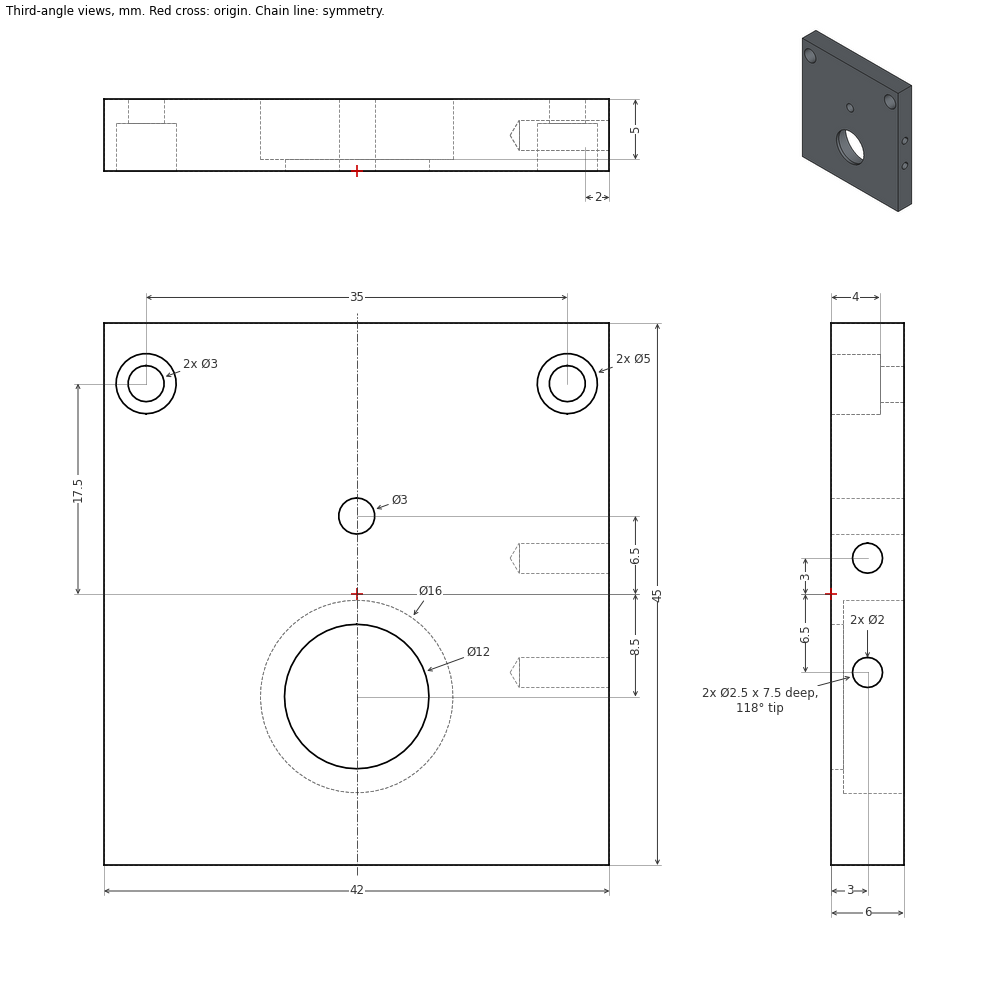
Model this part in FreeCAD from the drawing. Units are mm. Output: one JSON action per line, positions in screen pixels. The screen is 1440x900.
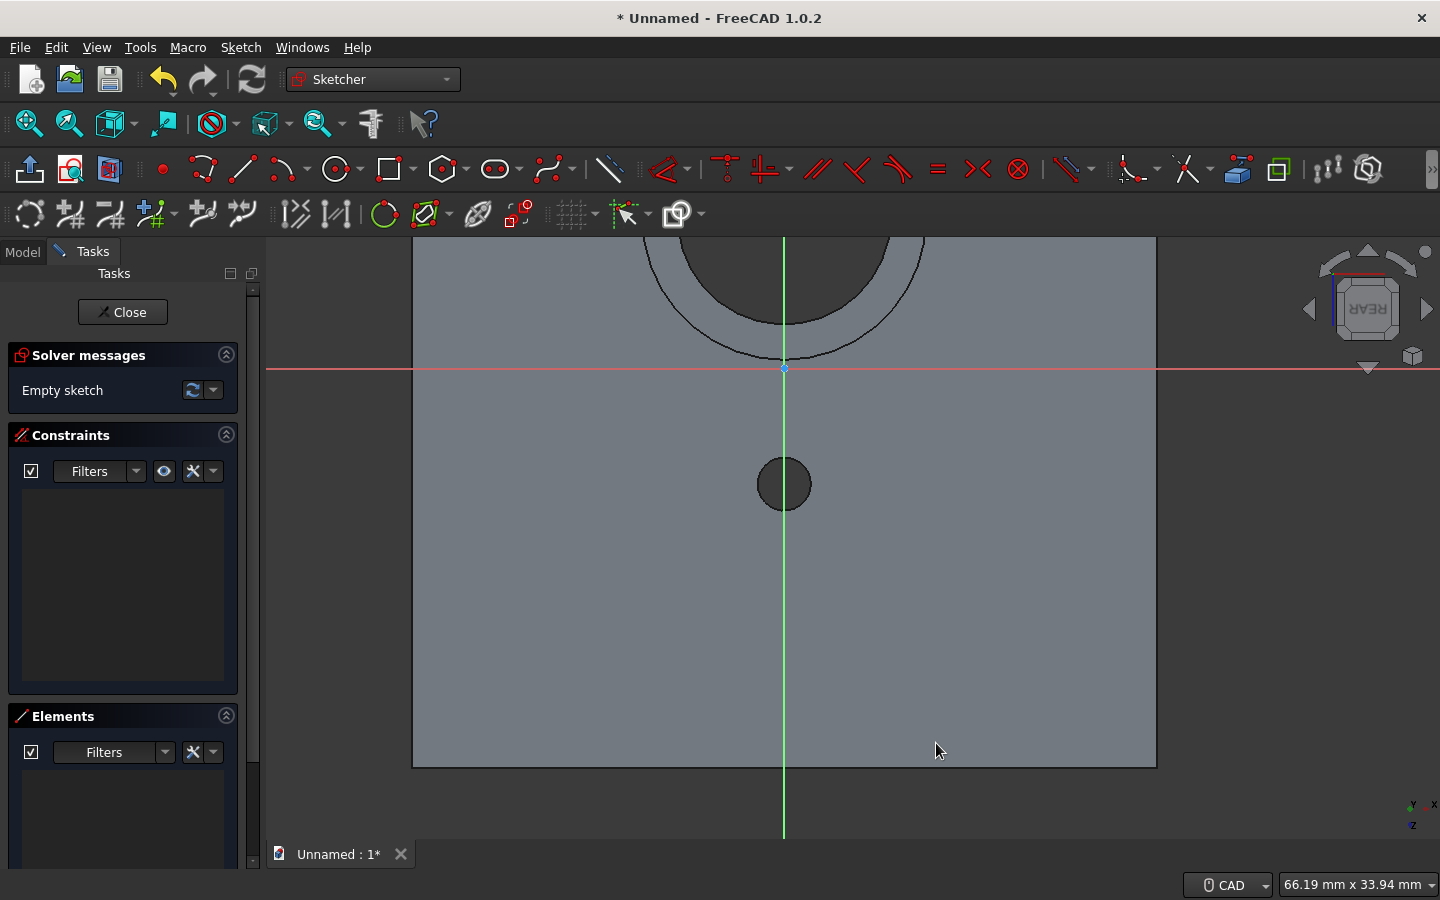
{"action": "key", "text": "g c"}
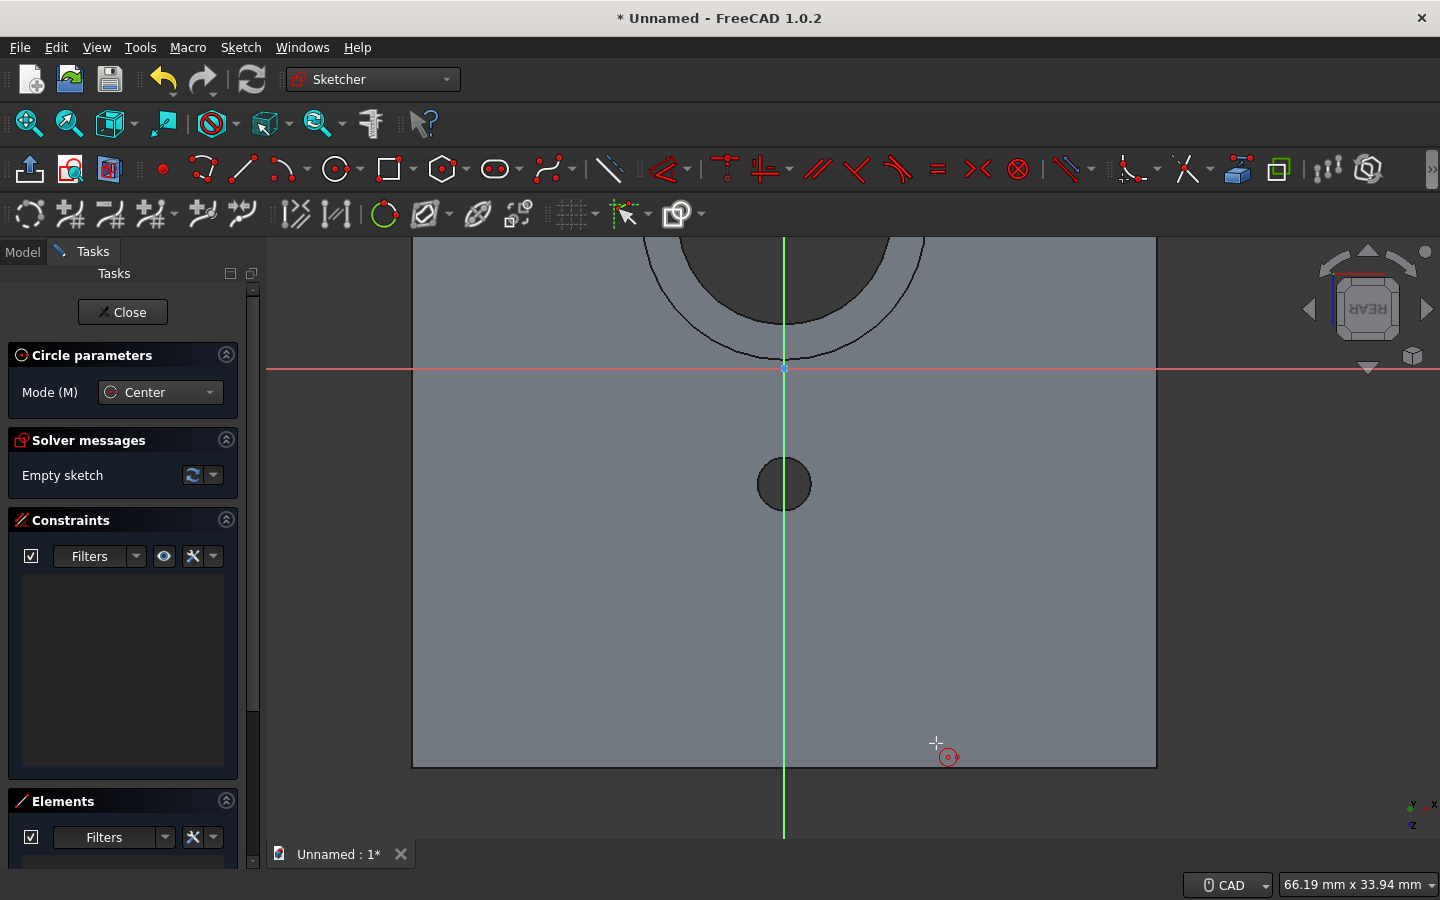
{"action": "left_click", "coordinate": [474, 679]}
{"action": "mouse_move", "coordinate": [493, 660]}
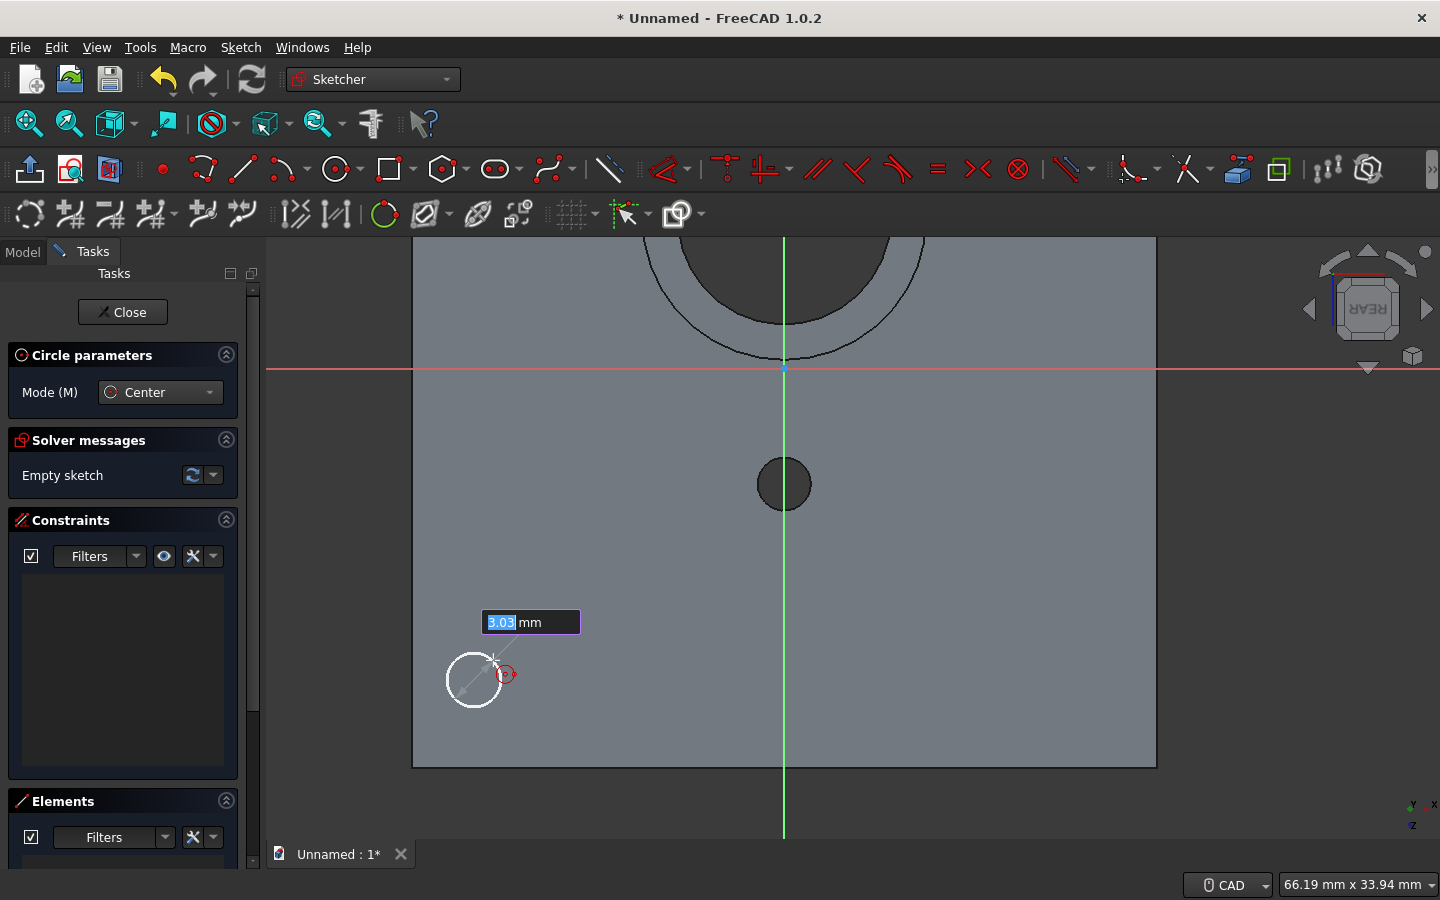
{"action": "type", "text": "3"}
{"action": "key", "text": "Return"}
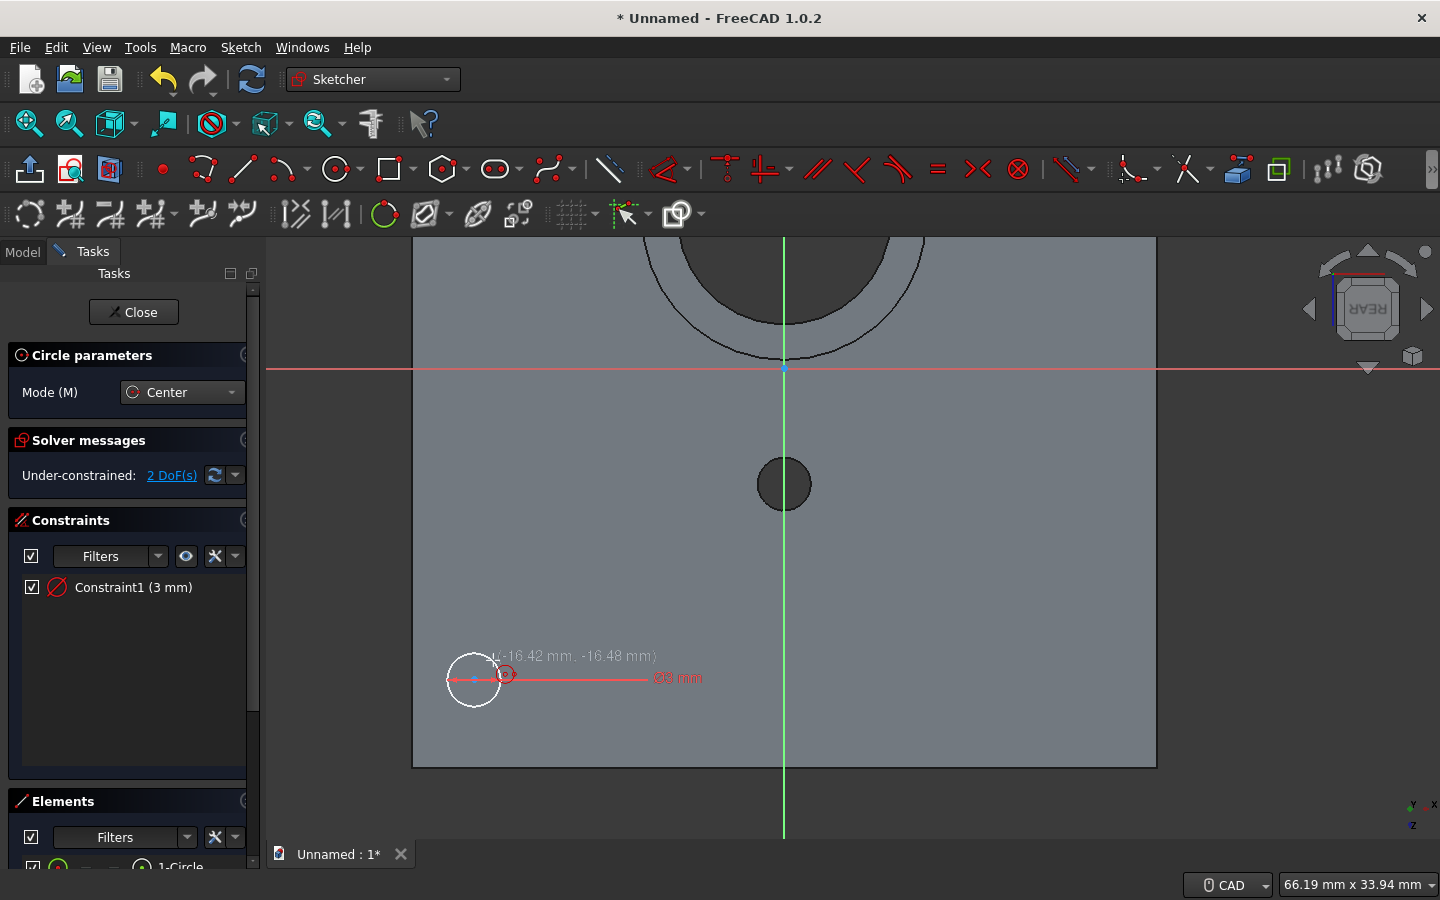
{"action": "left_click", "coordinate": [1095, 679]}
{"action": "mouse_move", "coordinate": [1113, 660]}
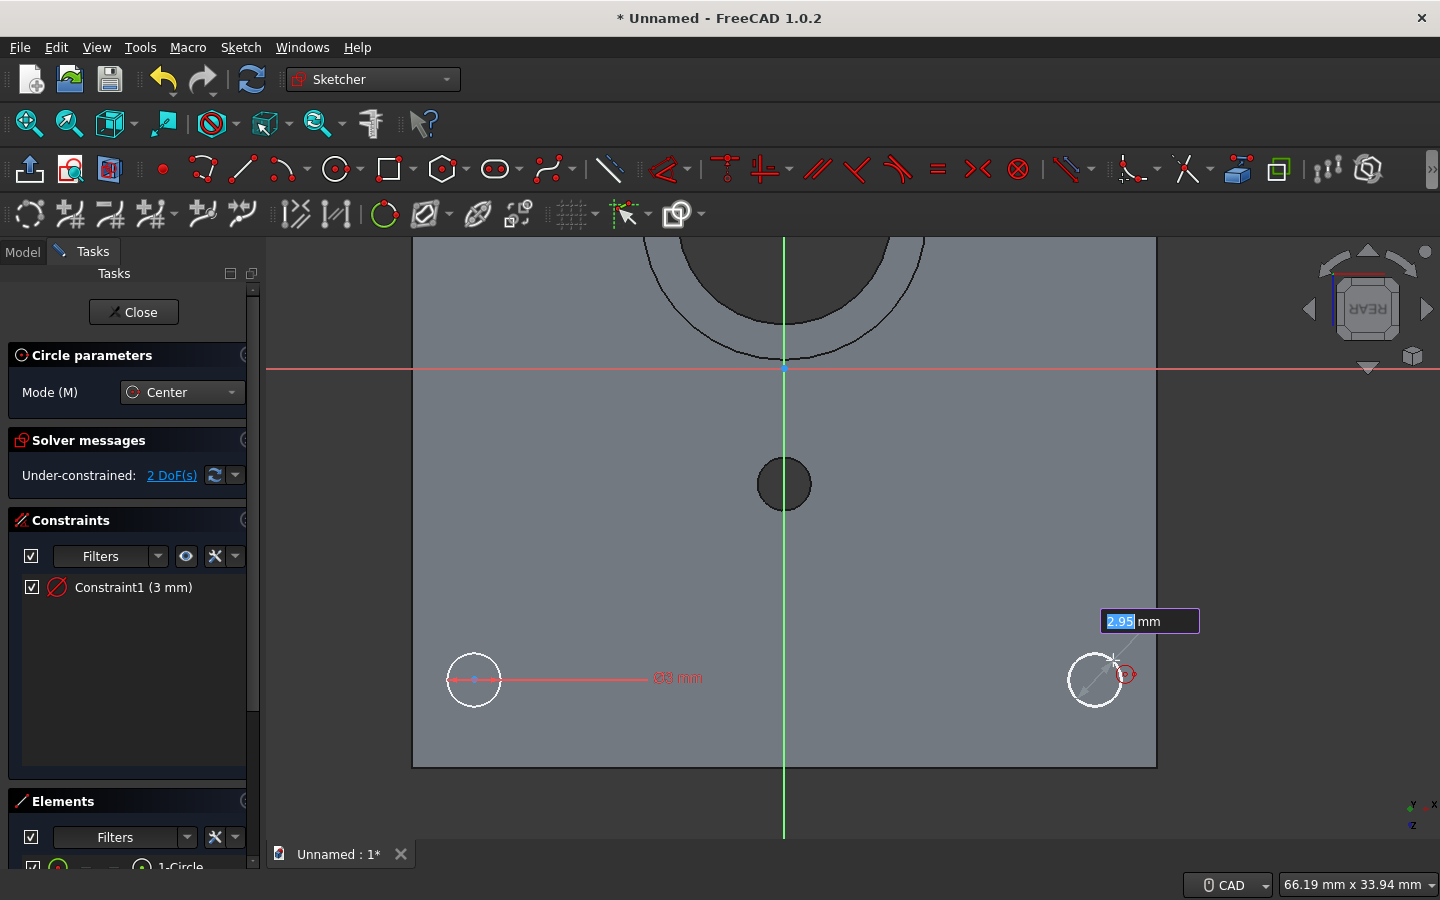
{"action": "type", "text": "3"}
{"action": "key", "text": "Return"}
{"action": "key", "text": "Escape"}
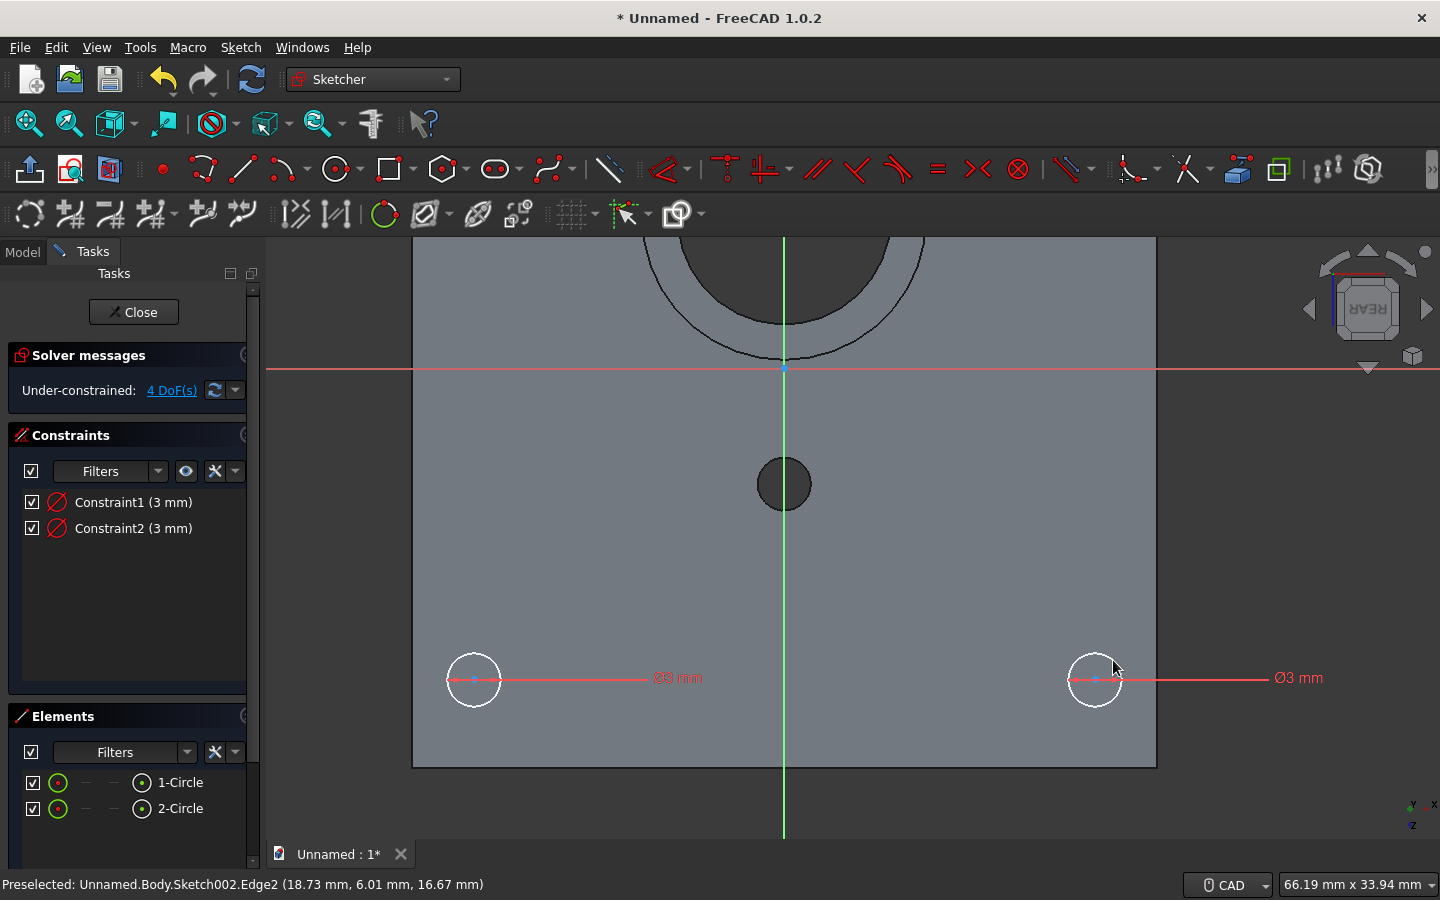
{"action": "left_click", "coordinate": [474, 680]}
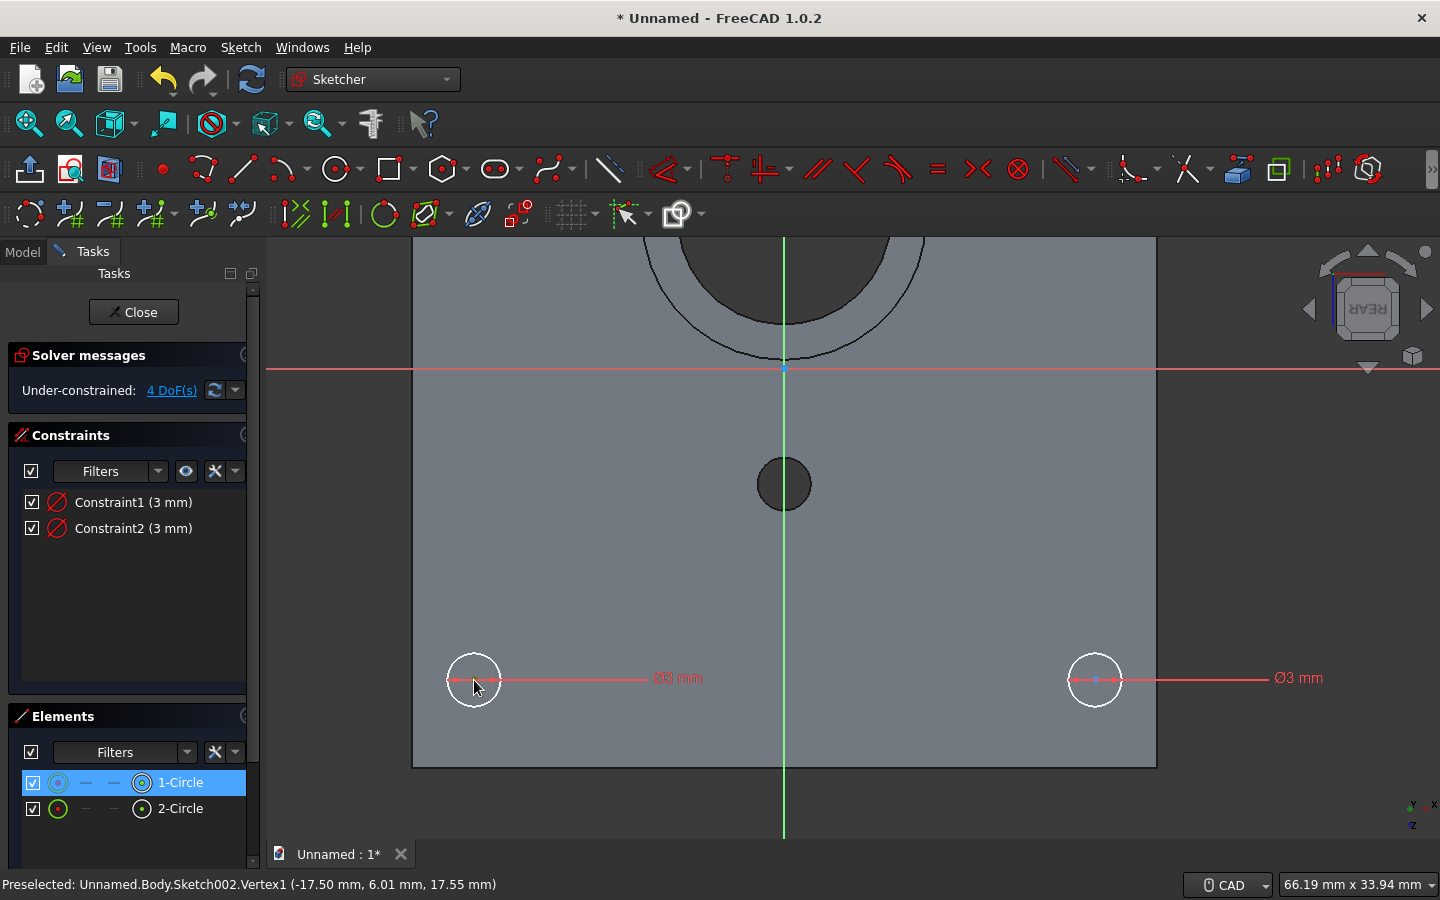
{"action": "left_click", "coordinate": [1095, 680]}